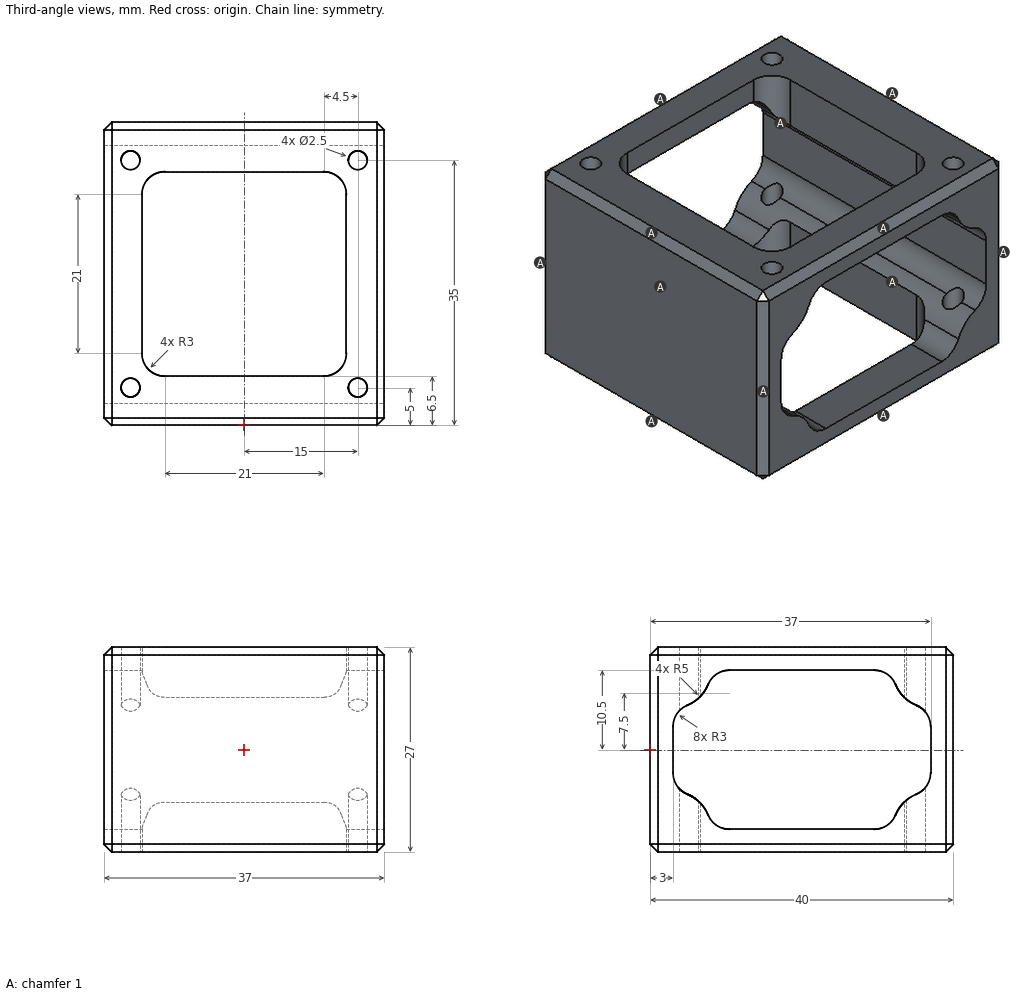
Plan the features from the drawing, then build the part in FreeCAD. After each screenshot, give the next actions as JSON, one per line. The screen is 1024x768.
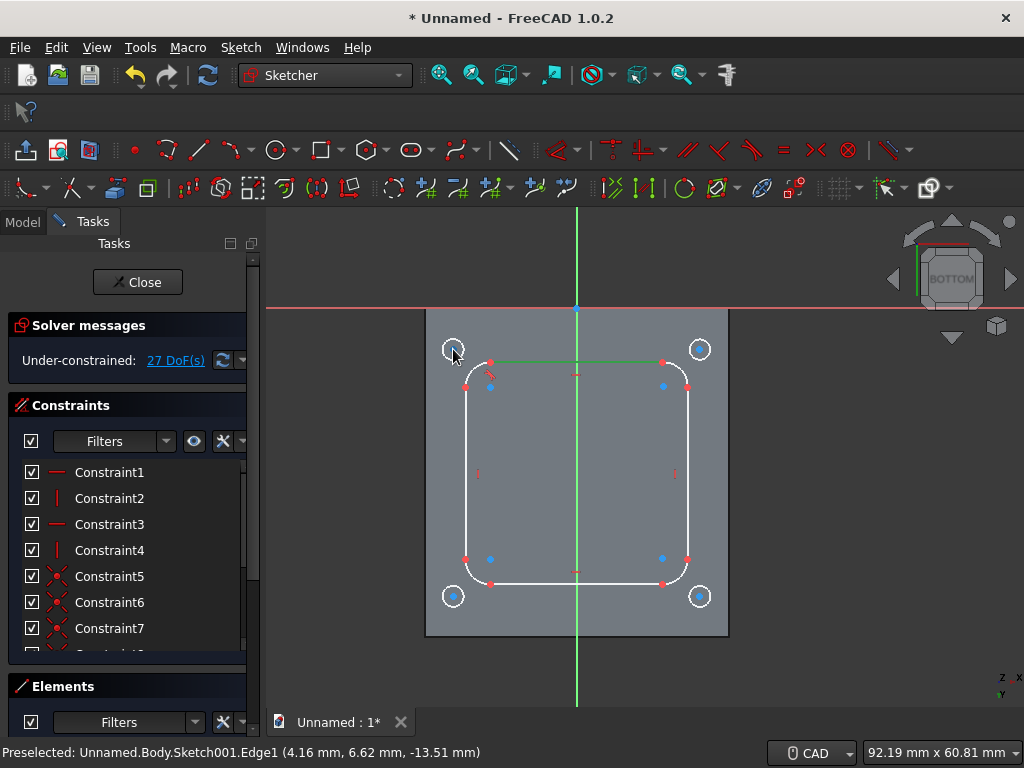
{"action": "left_click", "coordinate": [685, 376]}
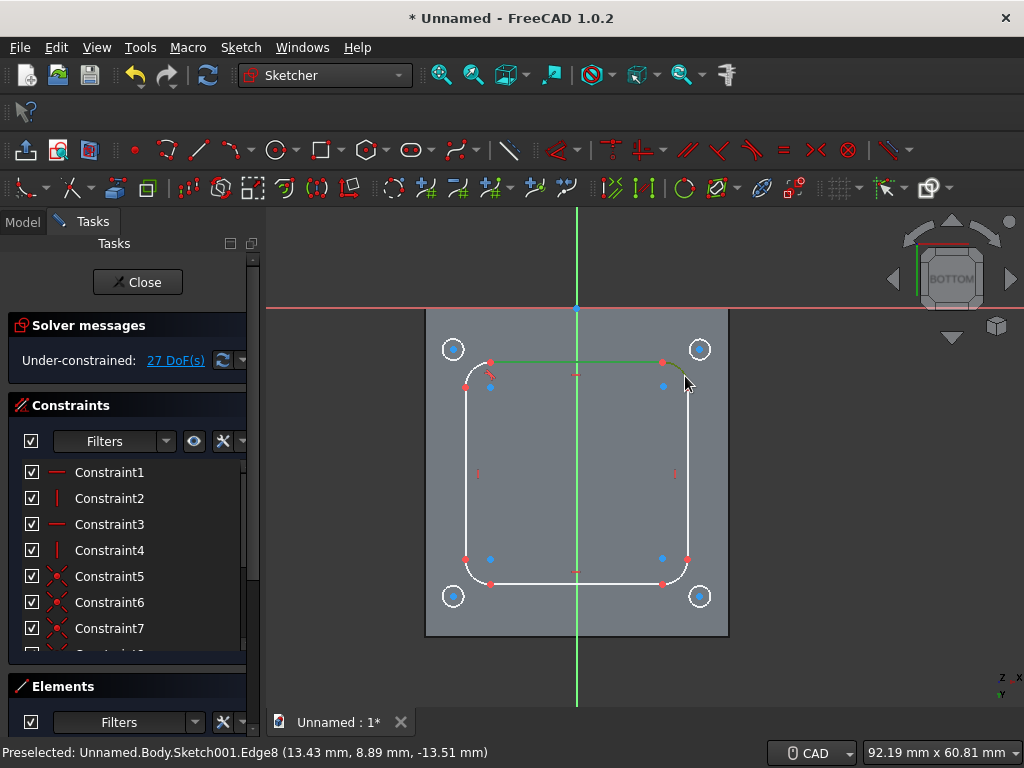
{"action": "key", "text": "t"}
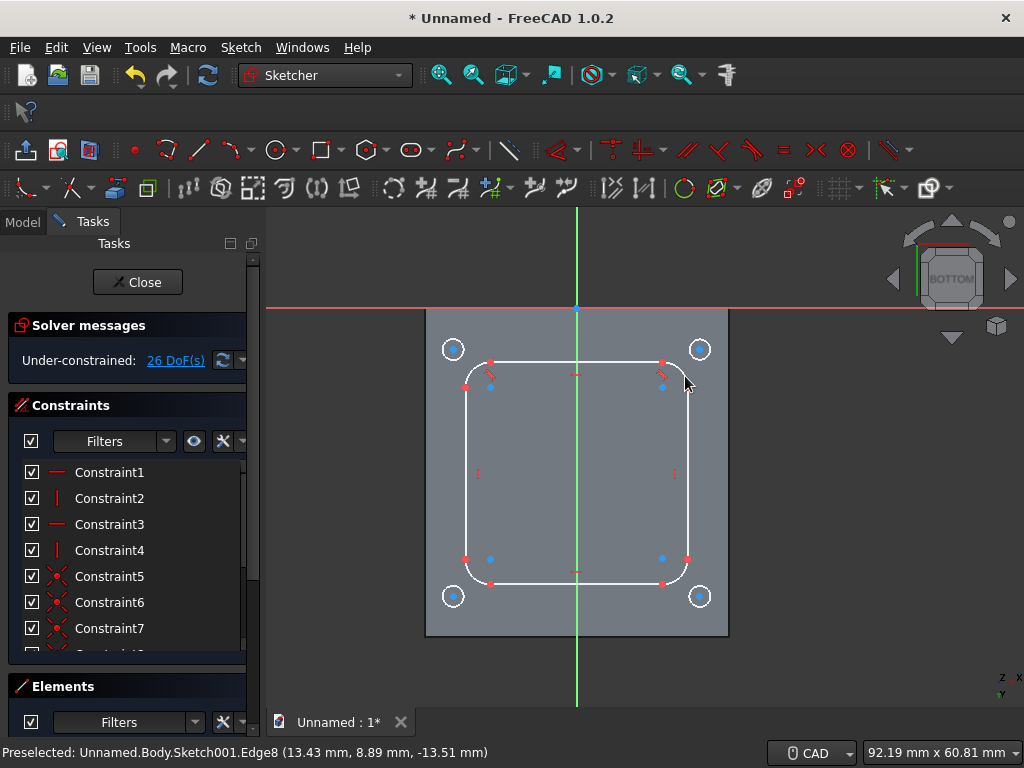
{"action": "left_click", "coordinate": [466, 439]}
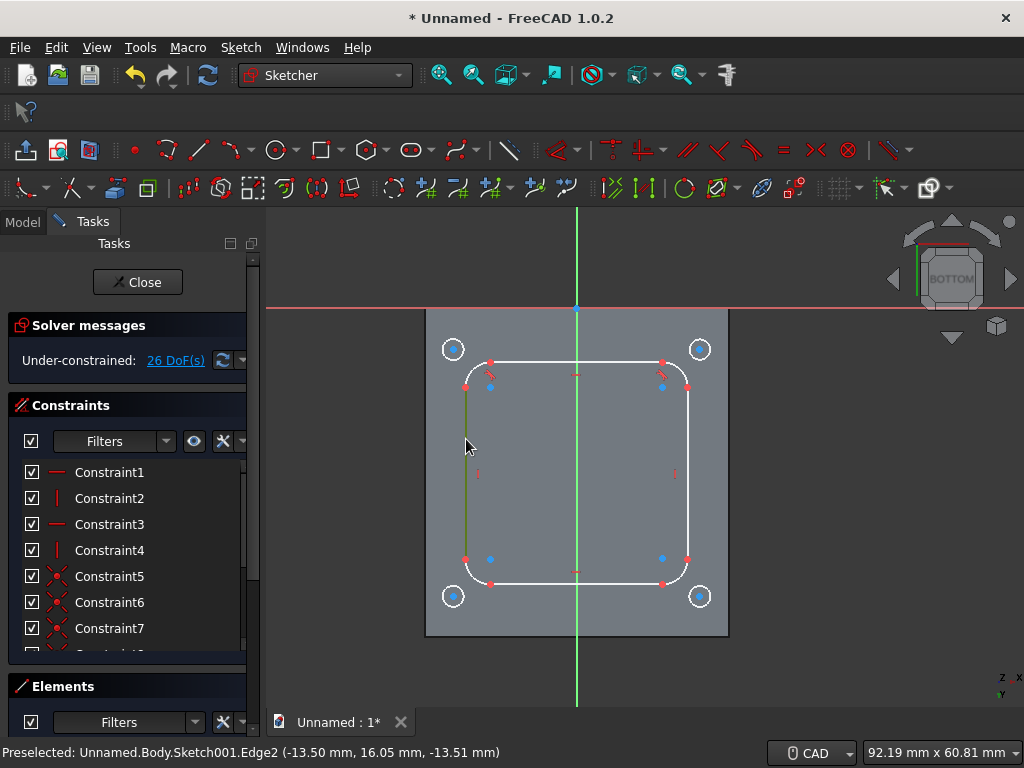
{"action": "left_click", "coordinate": [479, 365]}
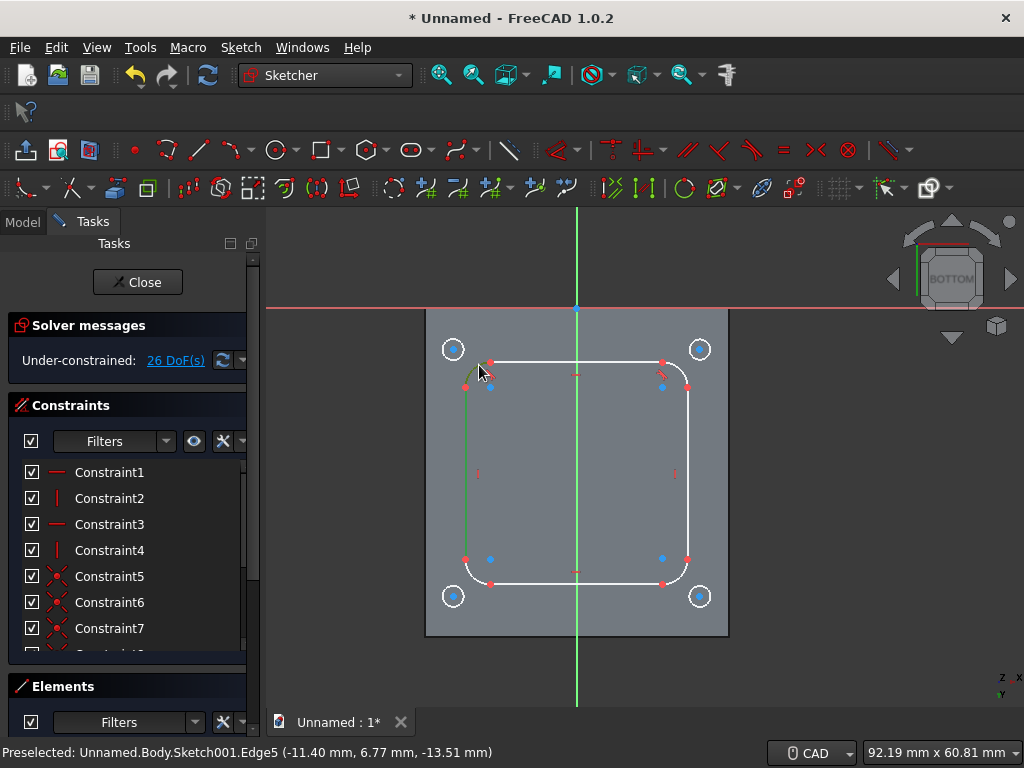
{"action": "left_click", "coordinate": [752, 150]}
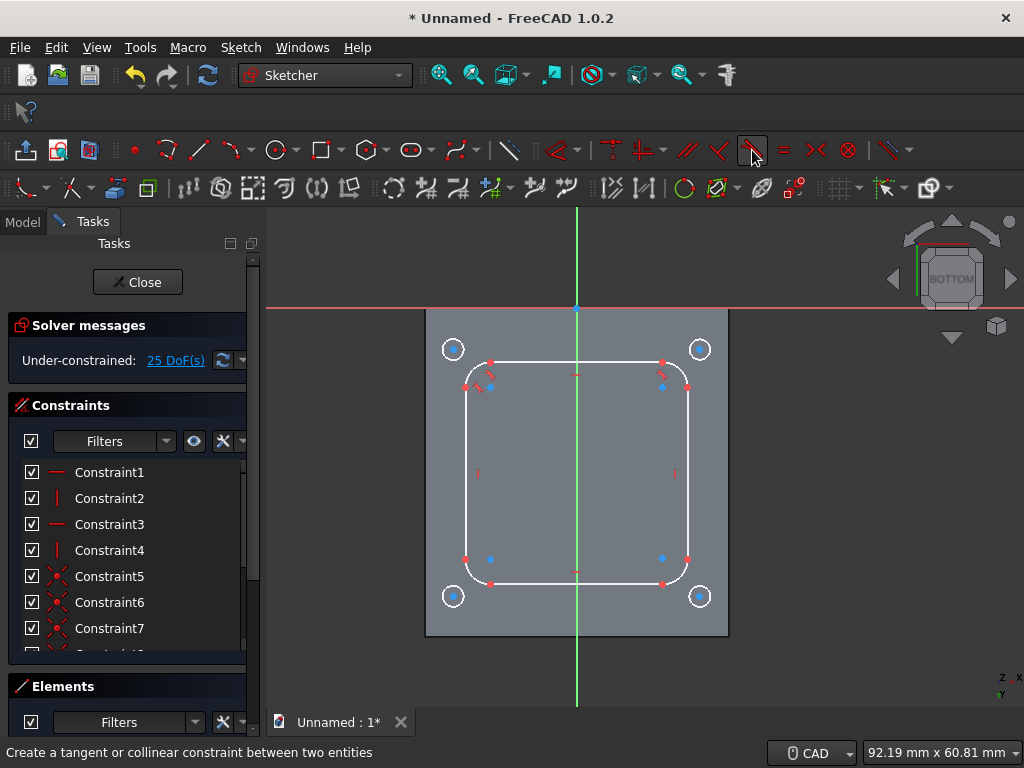
{"action": "left_click", "coordinate": [466, 439]}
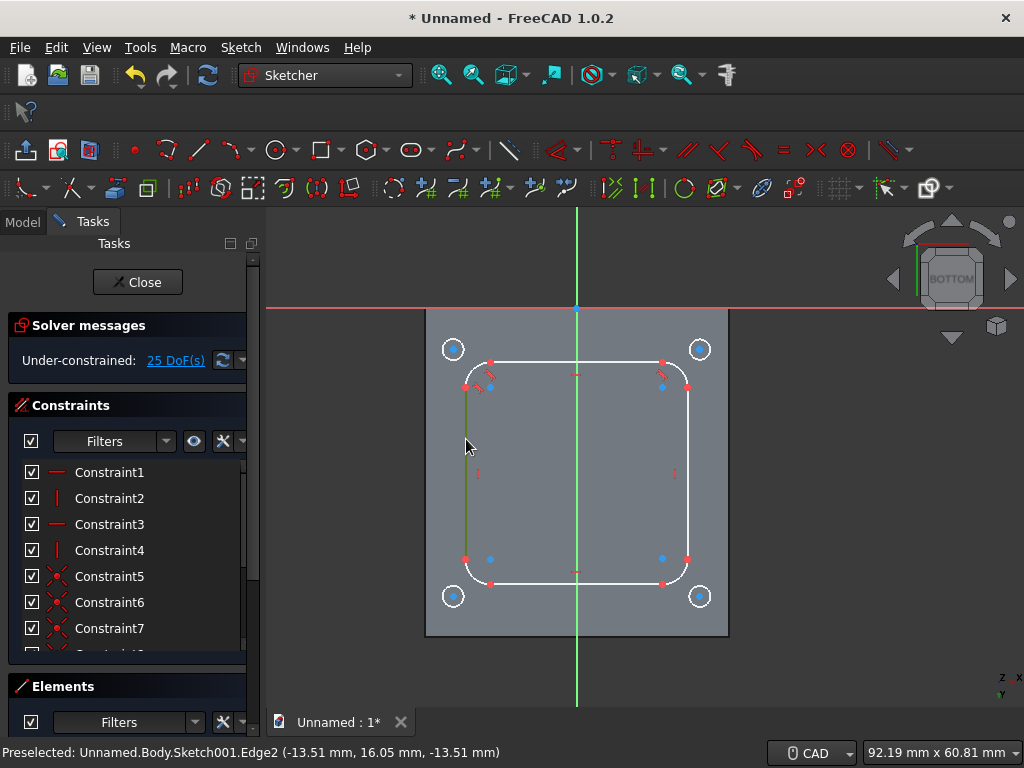
{"action": "left_click", "coordinate": [468, 571]}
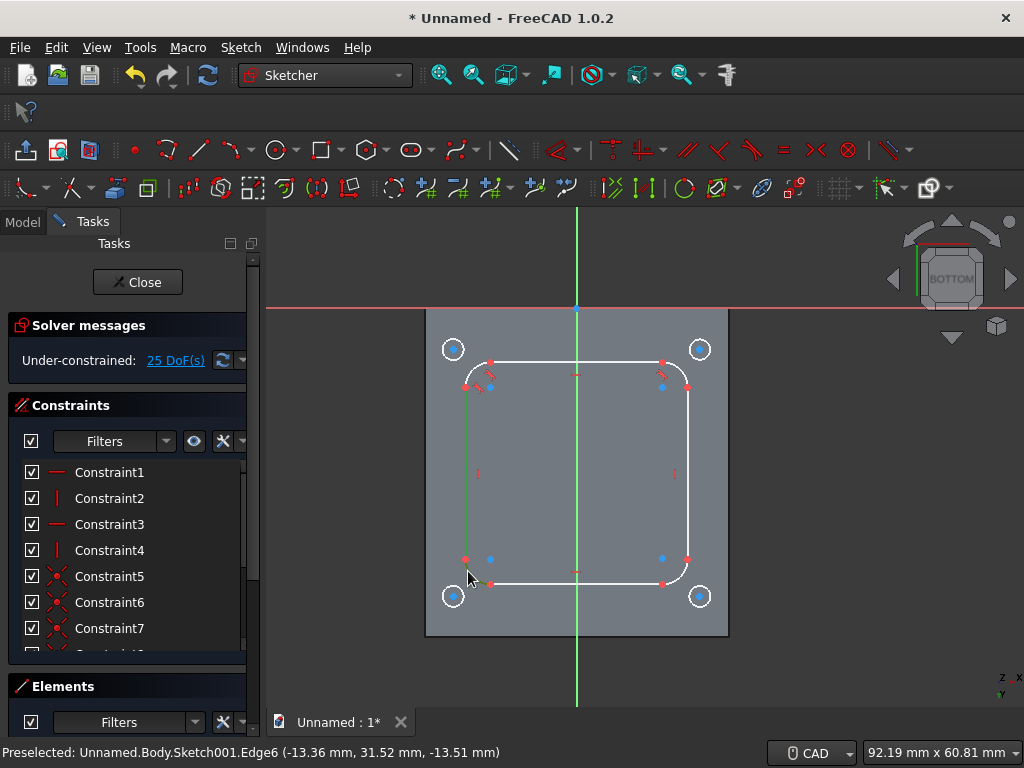
{"action": "key", "text": "t"}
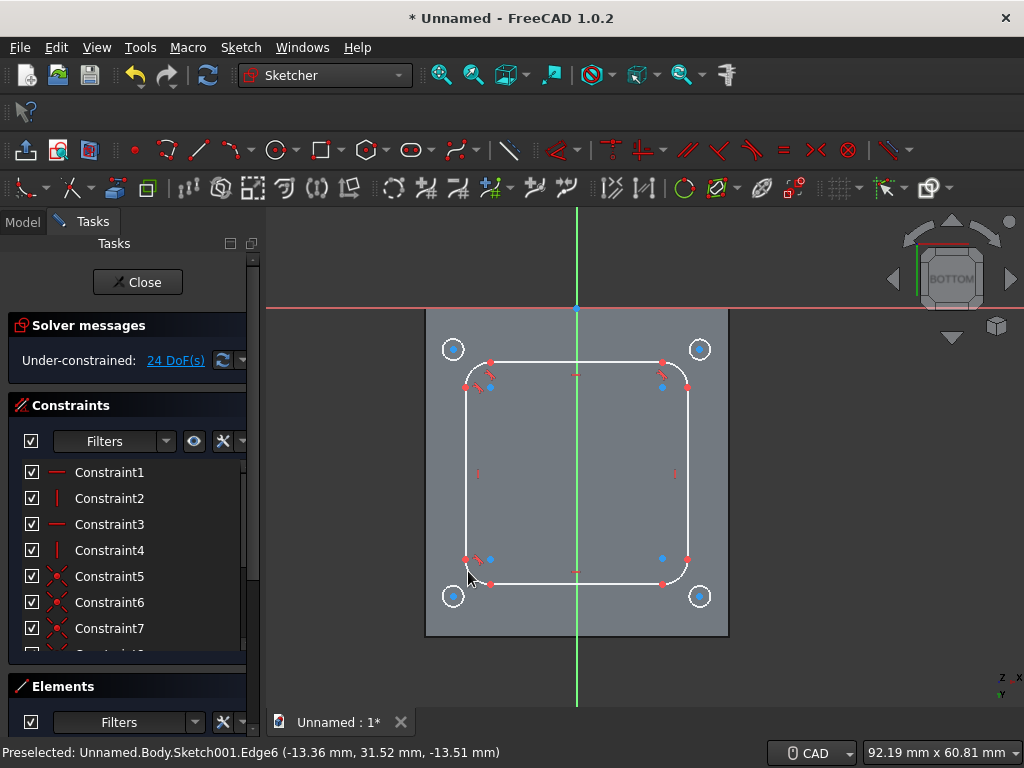
{"action": "left_click", "coordinate": [542, 584]}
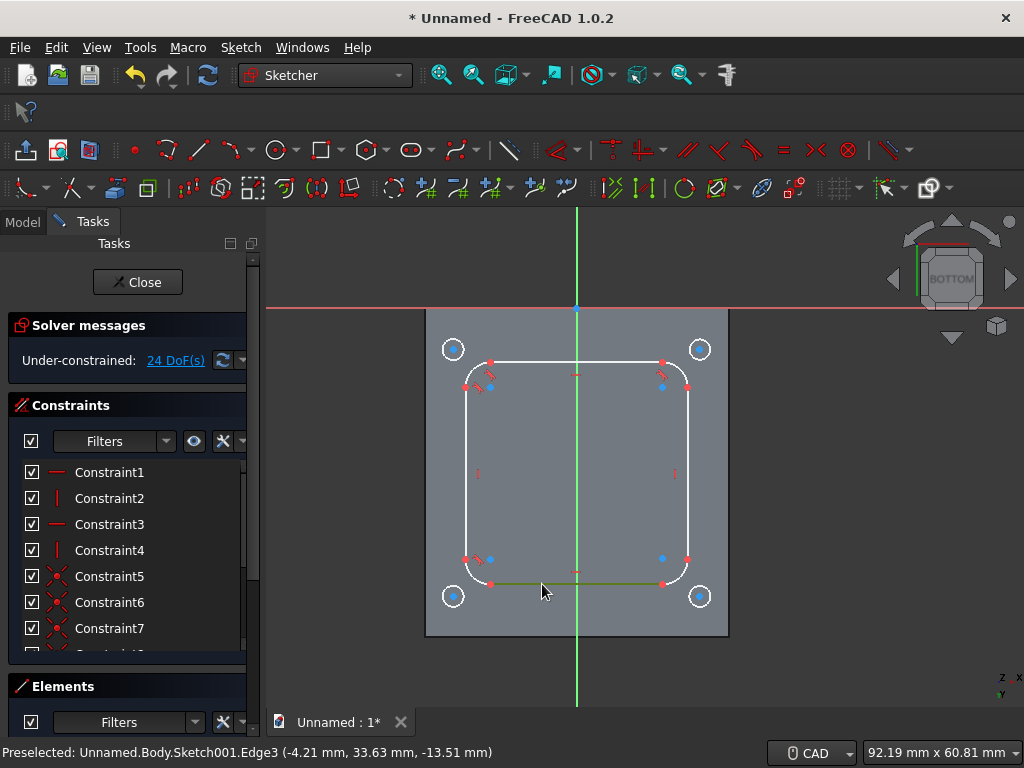
{"action": "left_click", "coordinate": [468, 571]}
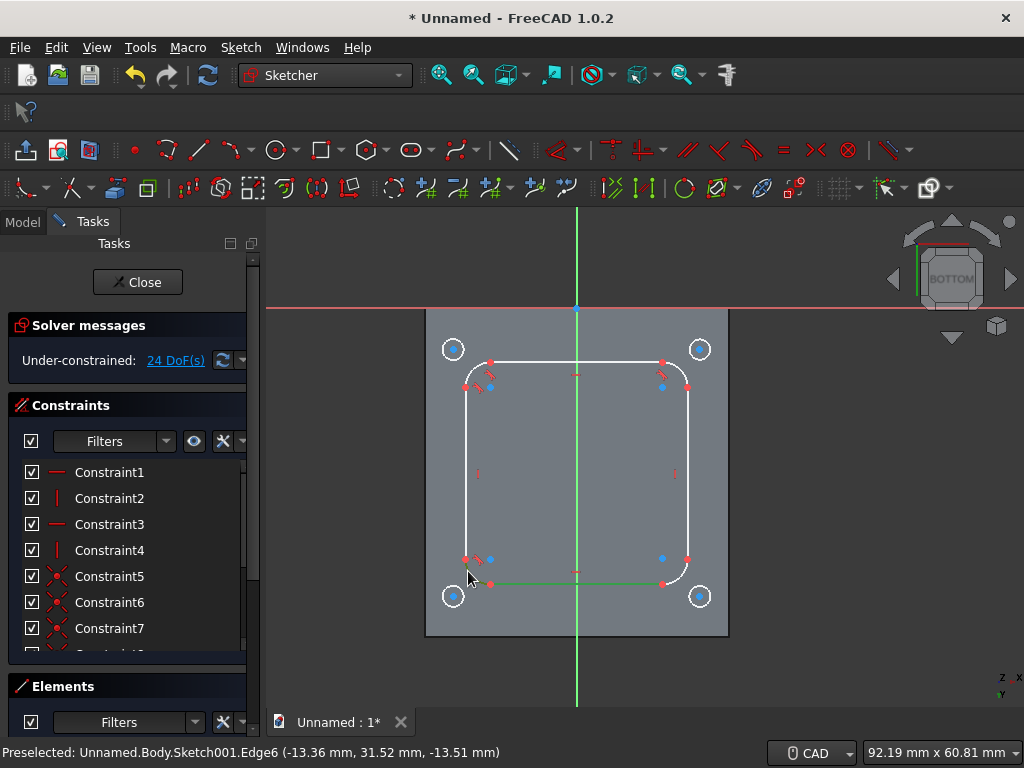
{"action": "key", "text": "t"}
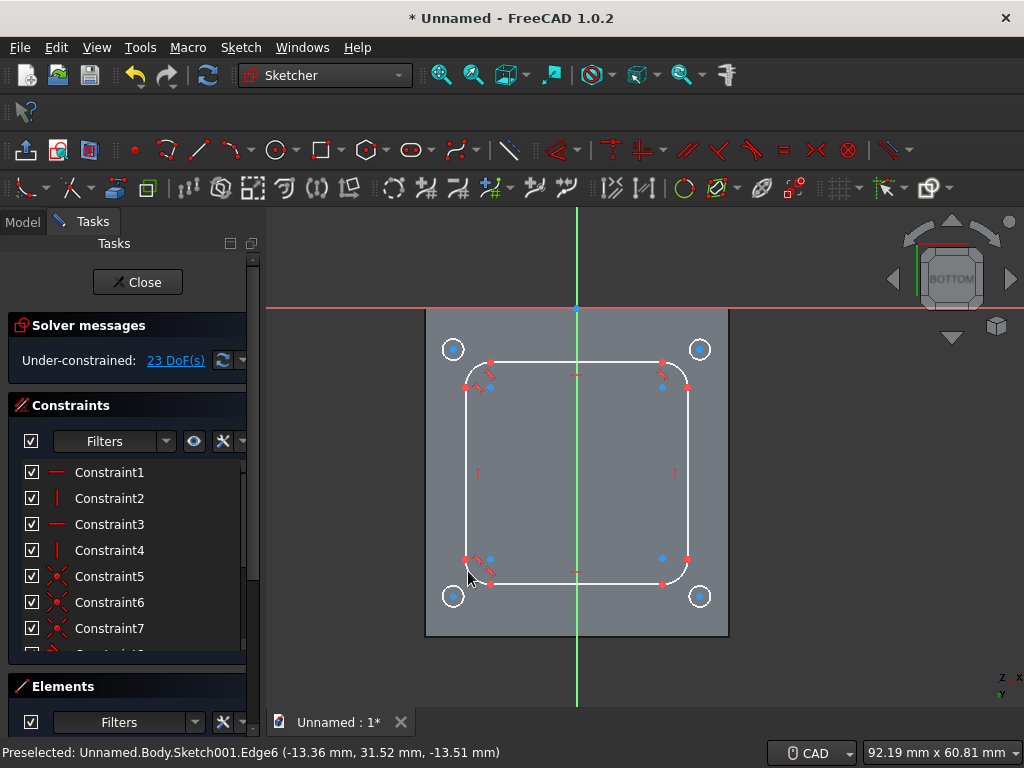
{"action": "left_click", "coordinate": [542, 584]}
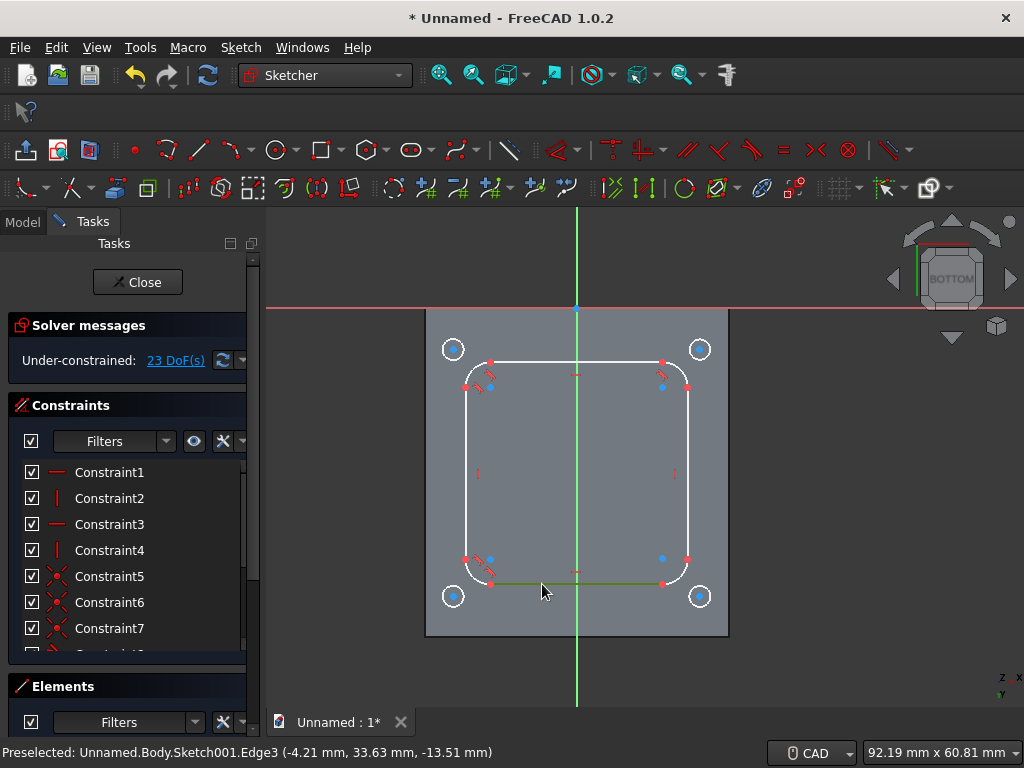
{"action": "left_click", "coordinate": [674, 582]}